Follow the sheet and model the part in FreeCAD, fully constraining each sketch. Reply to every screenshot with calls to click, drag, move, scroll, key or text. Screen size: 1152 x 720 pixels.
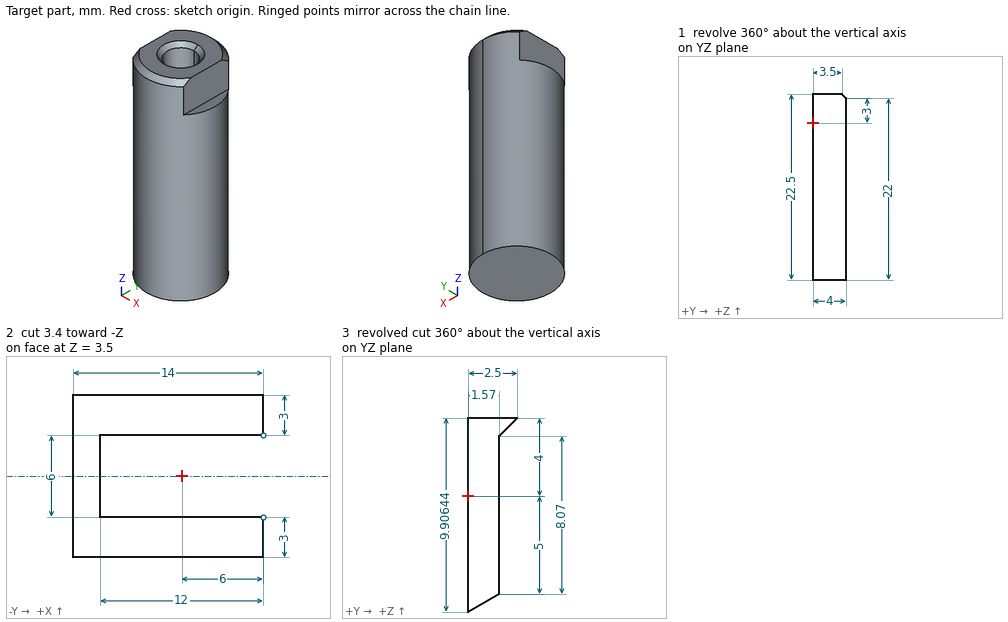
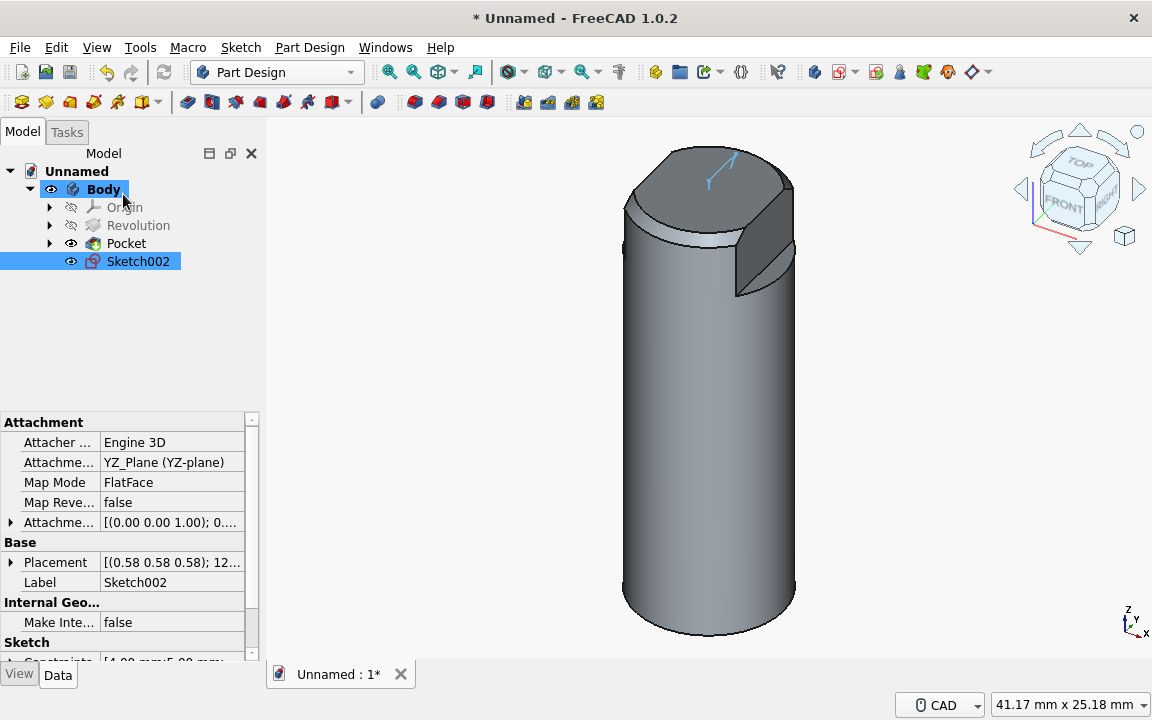
click(236, 102)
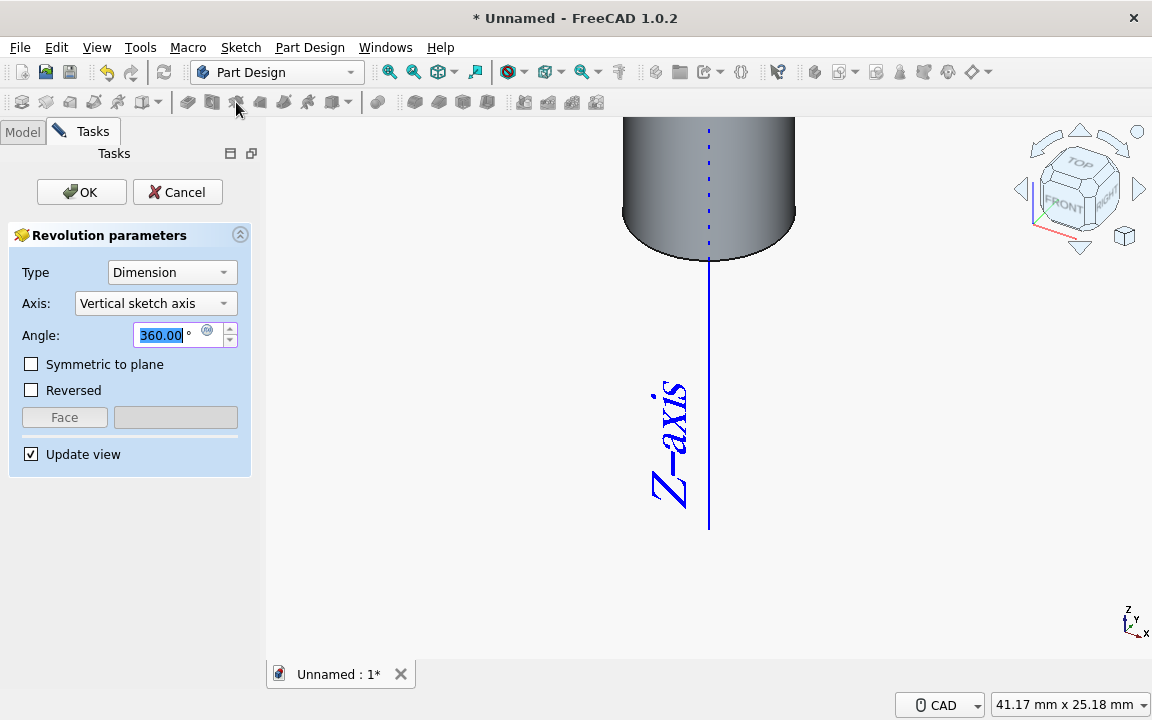
click(82, 192)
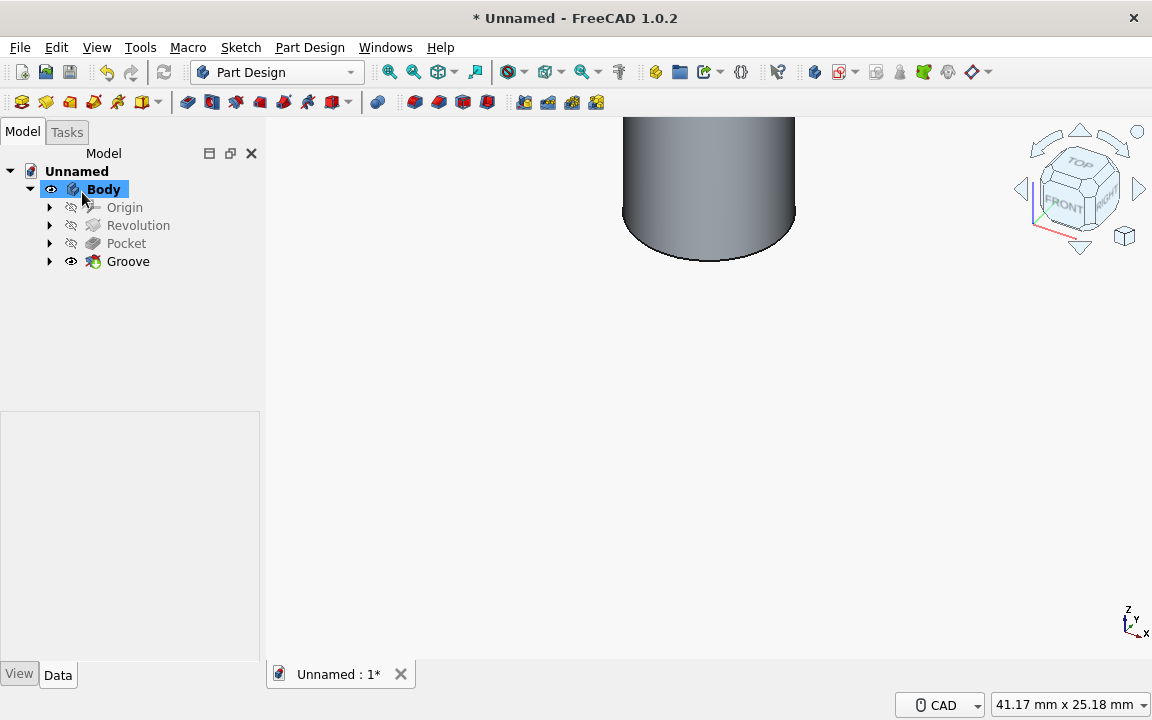
key(0)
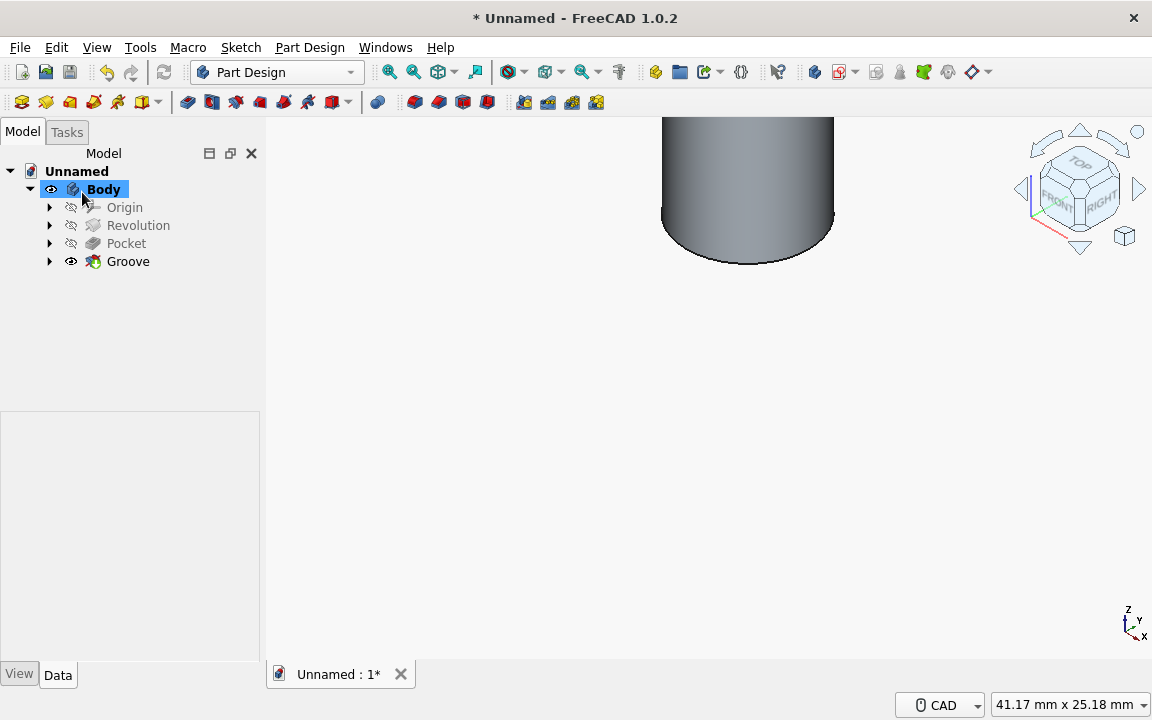
click(390, 72)